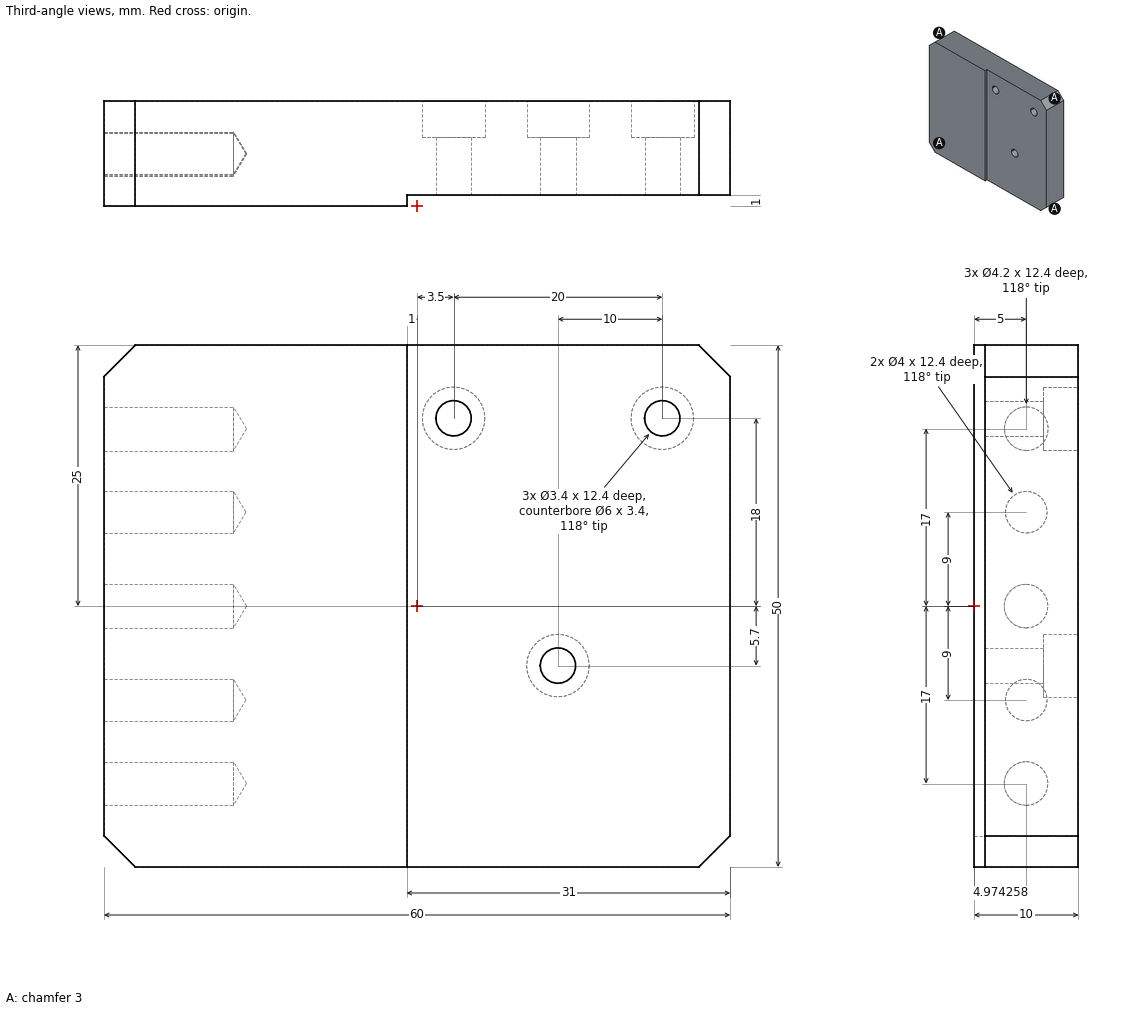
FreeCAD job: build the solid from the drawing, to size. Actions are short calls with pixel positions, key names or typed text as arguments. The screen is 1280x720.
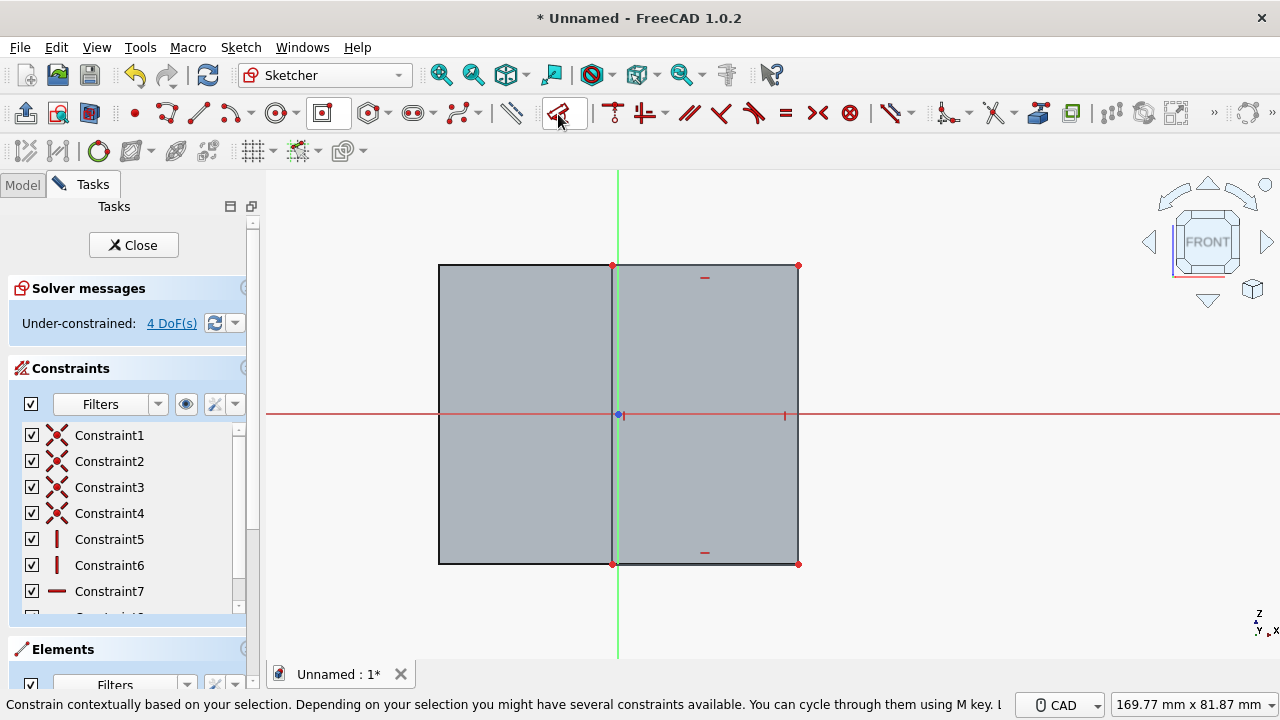
scroll(612, 355, up, 5)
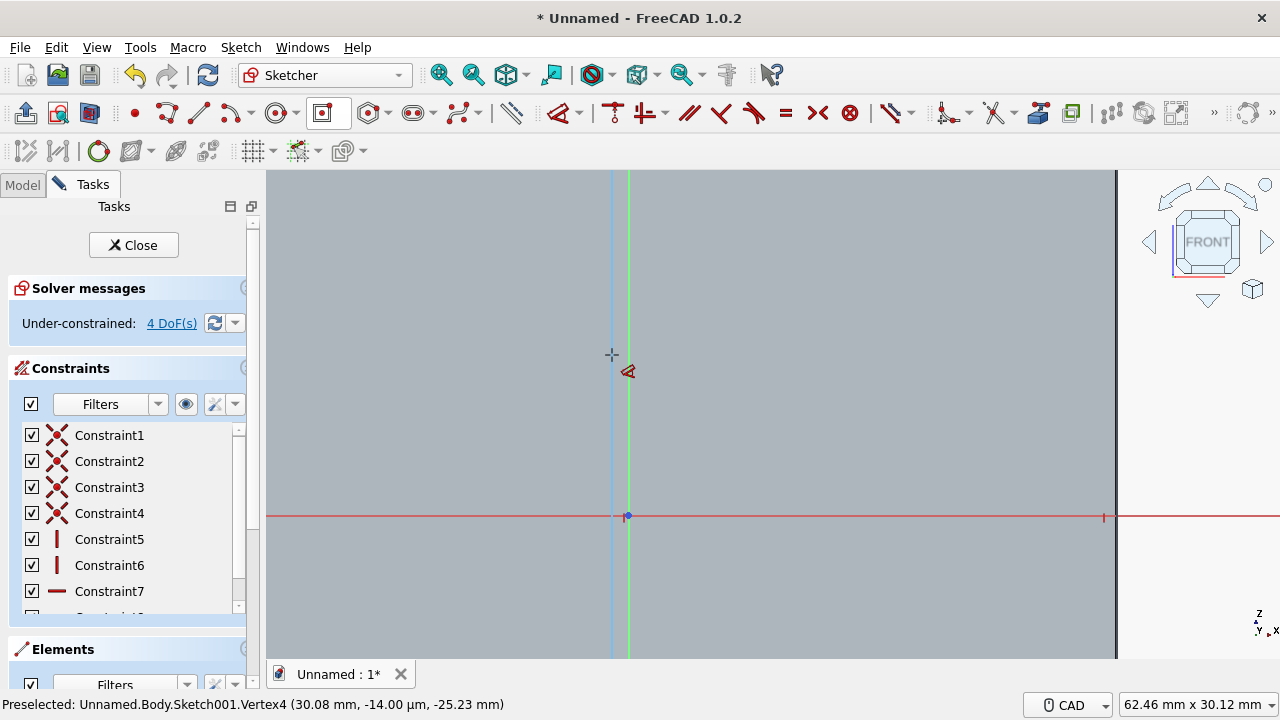
click(612, 355)
click(578, 414)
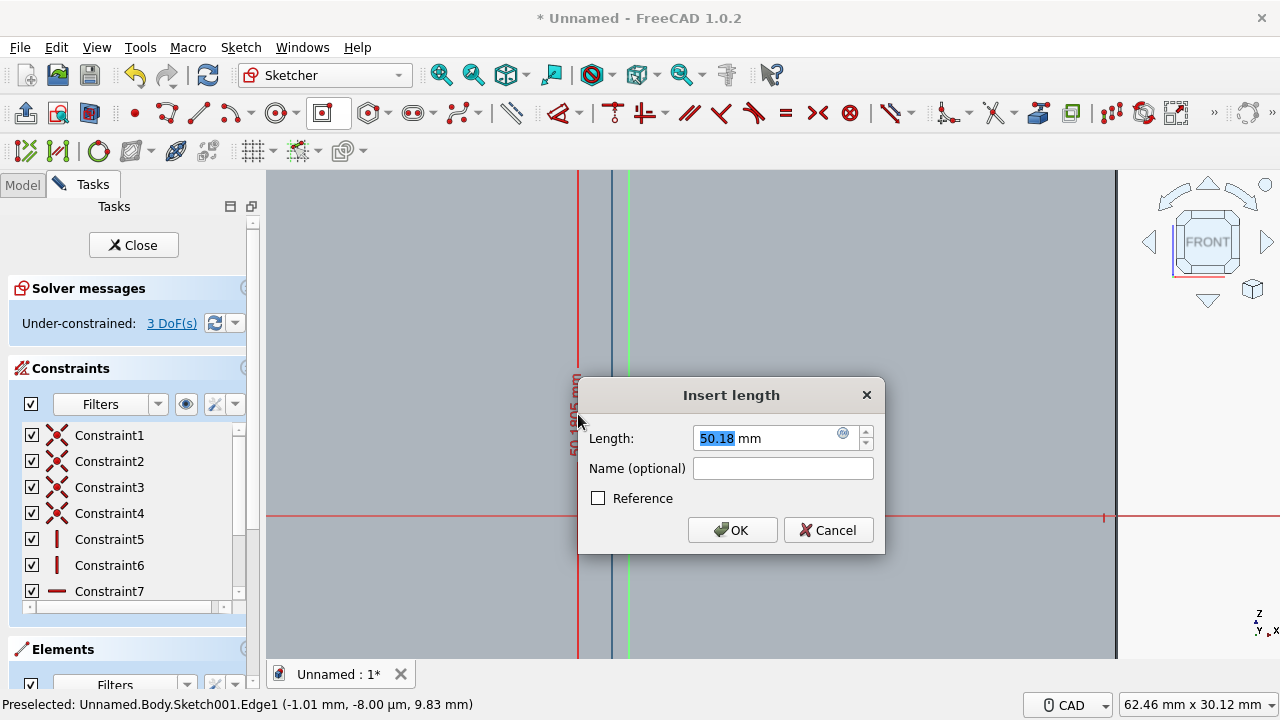
text(50)
key(Return)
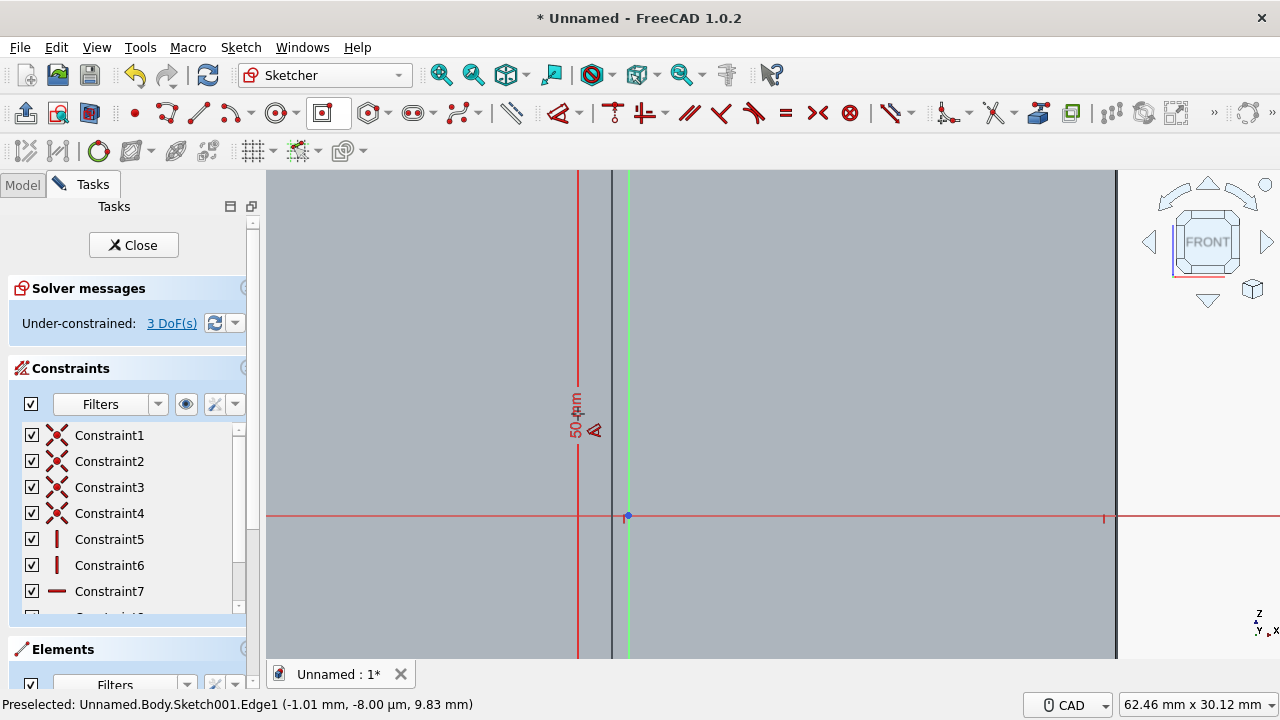
scroll(612, 356, down, 5)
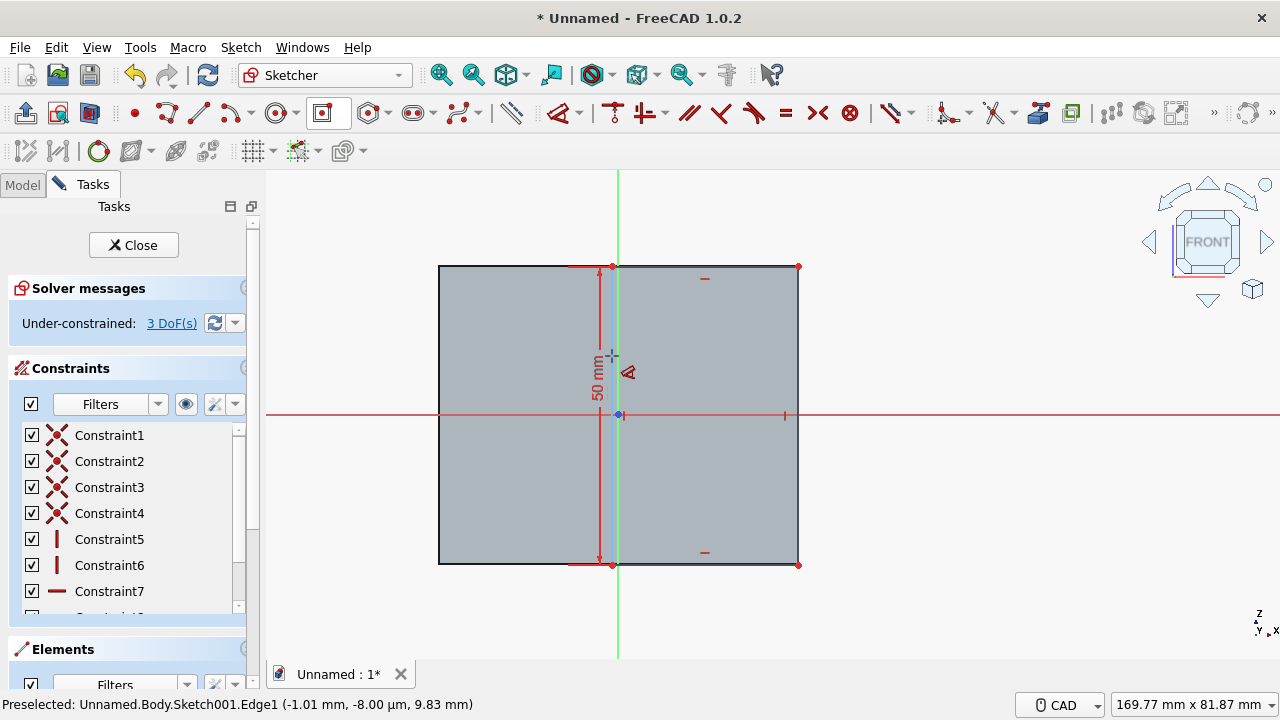
click(668, 565)
click(705, 599)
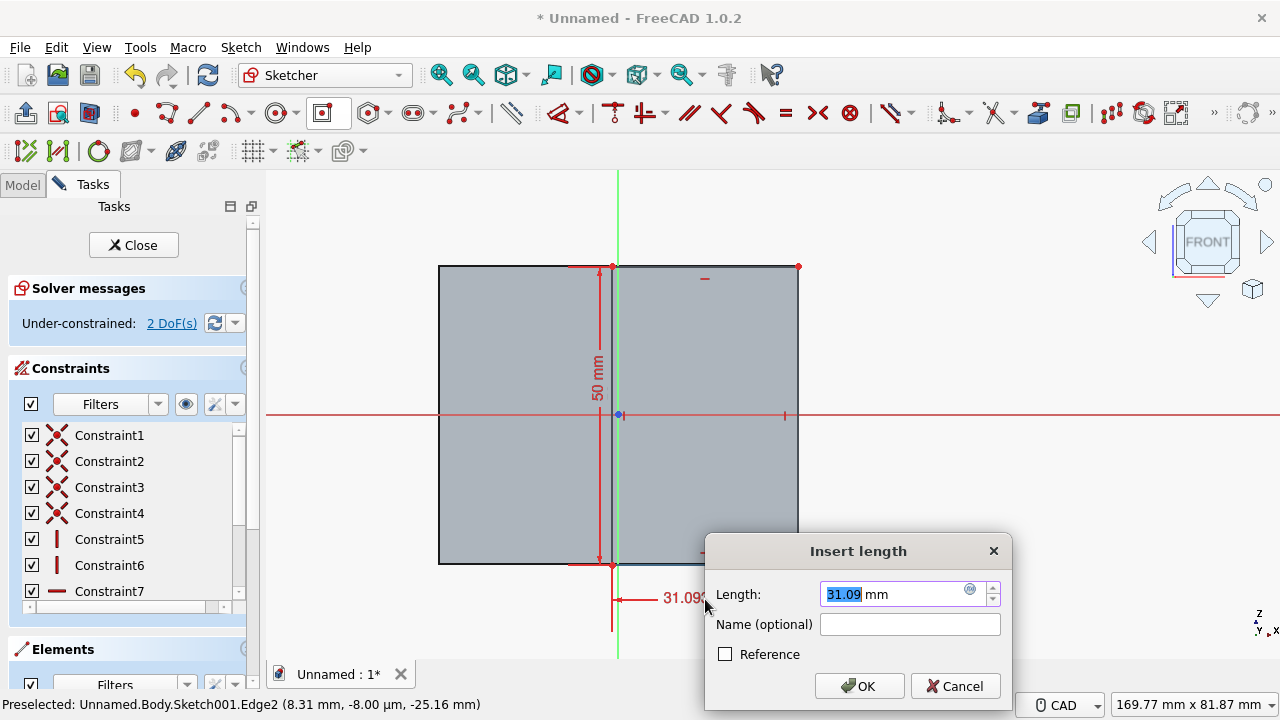
text(31)
key(Return)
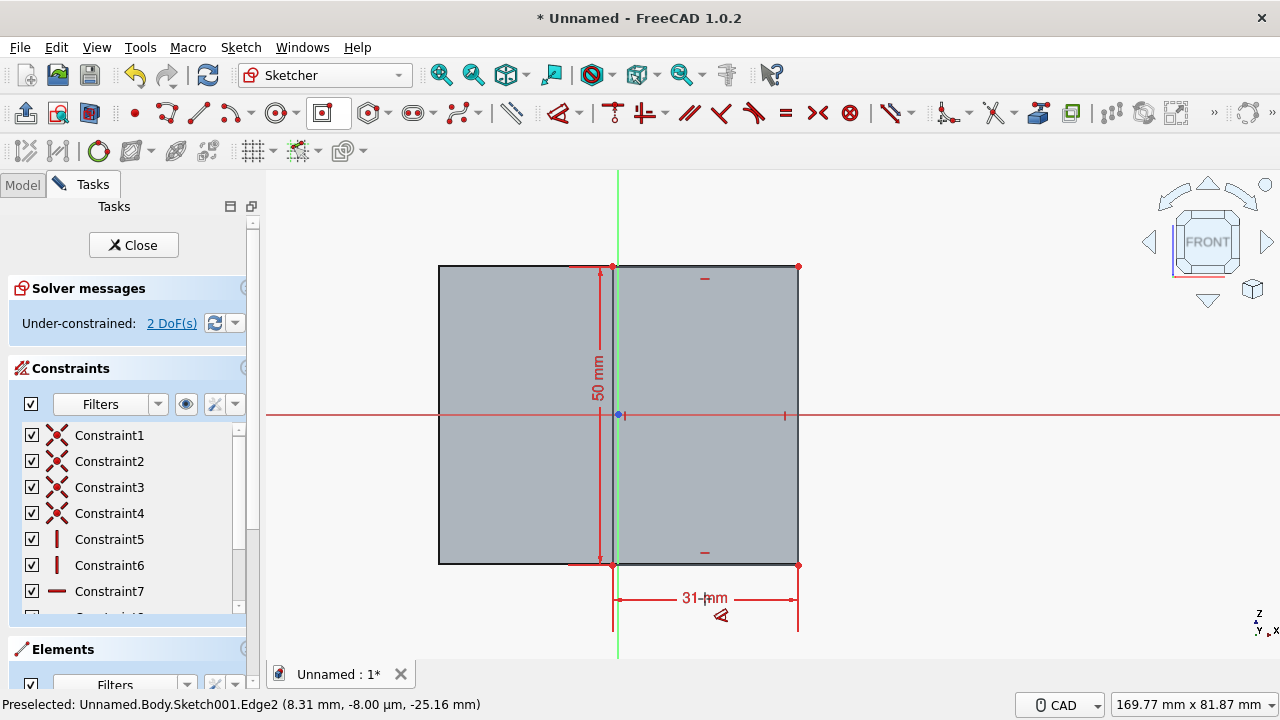
scroll(613, 267, up, 10)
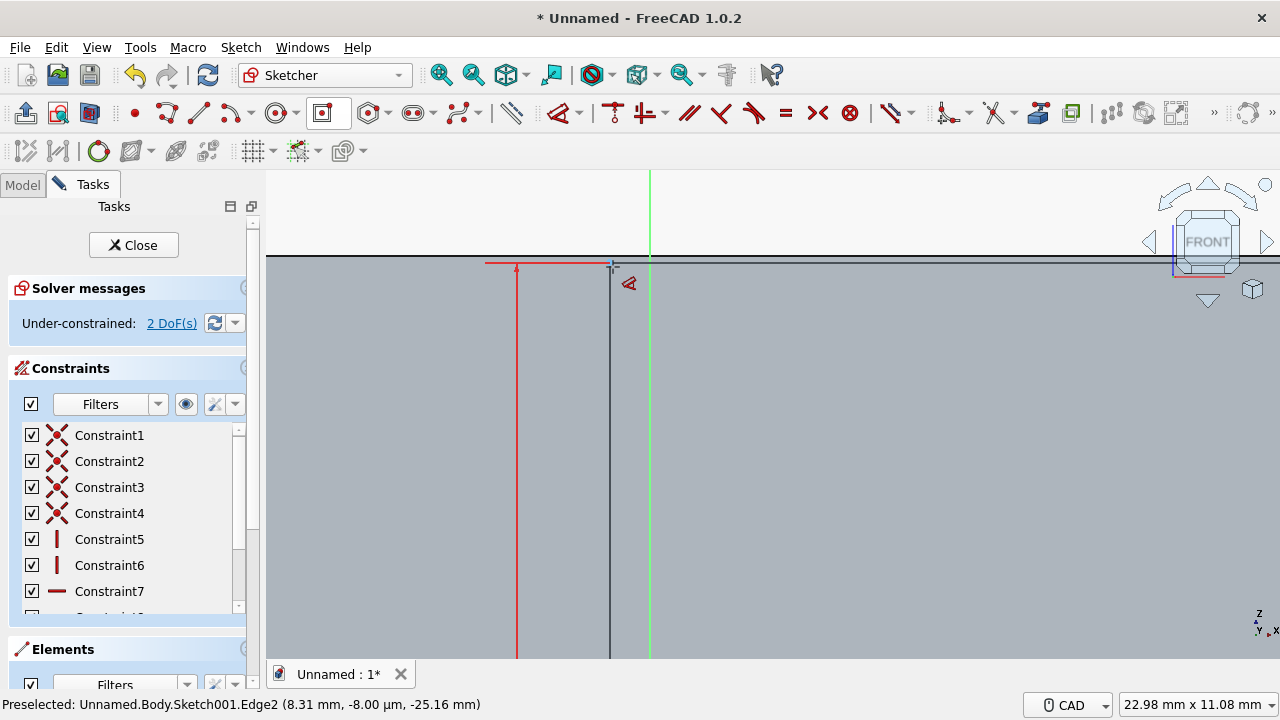
click(610, 263)
click(630, 229)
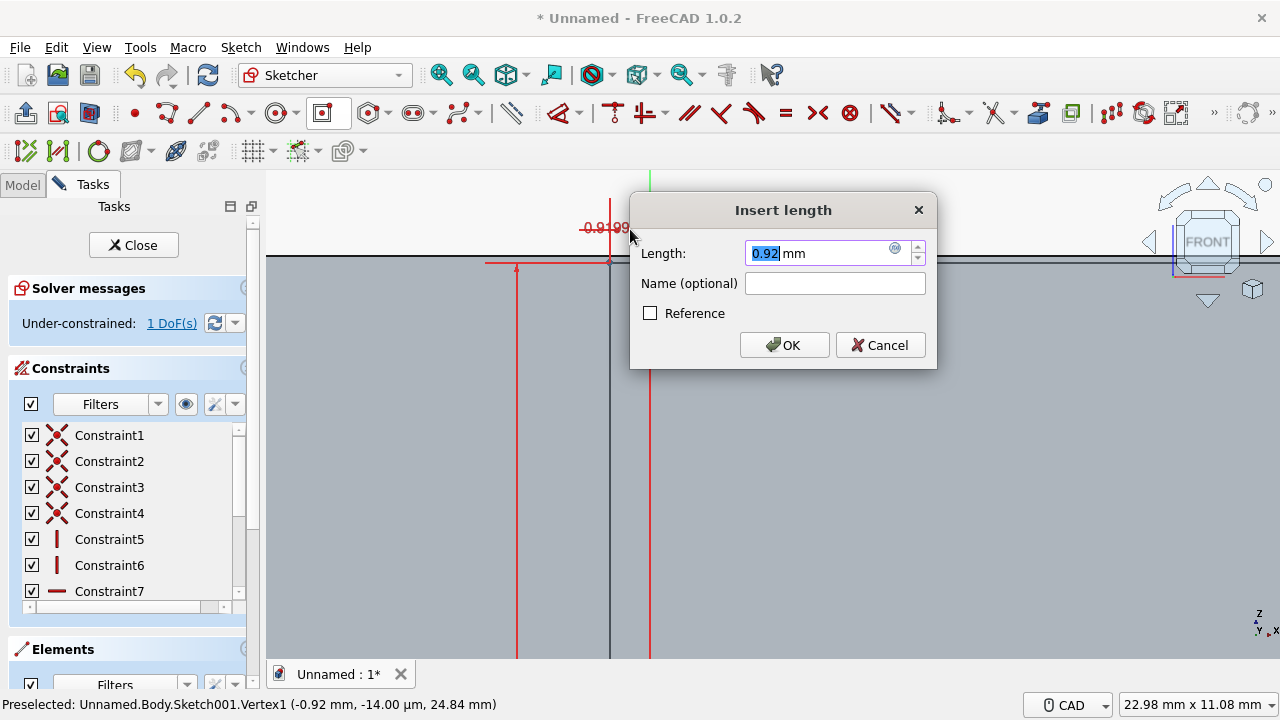
text(1)
key(Return)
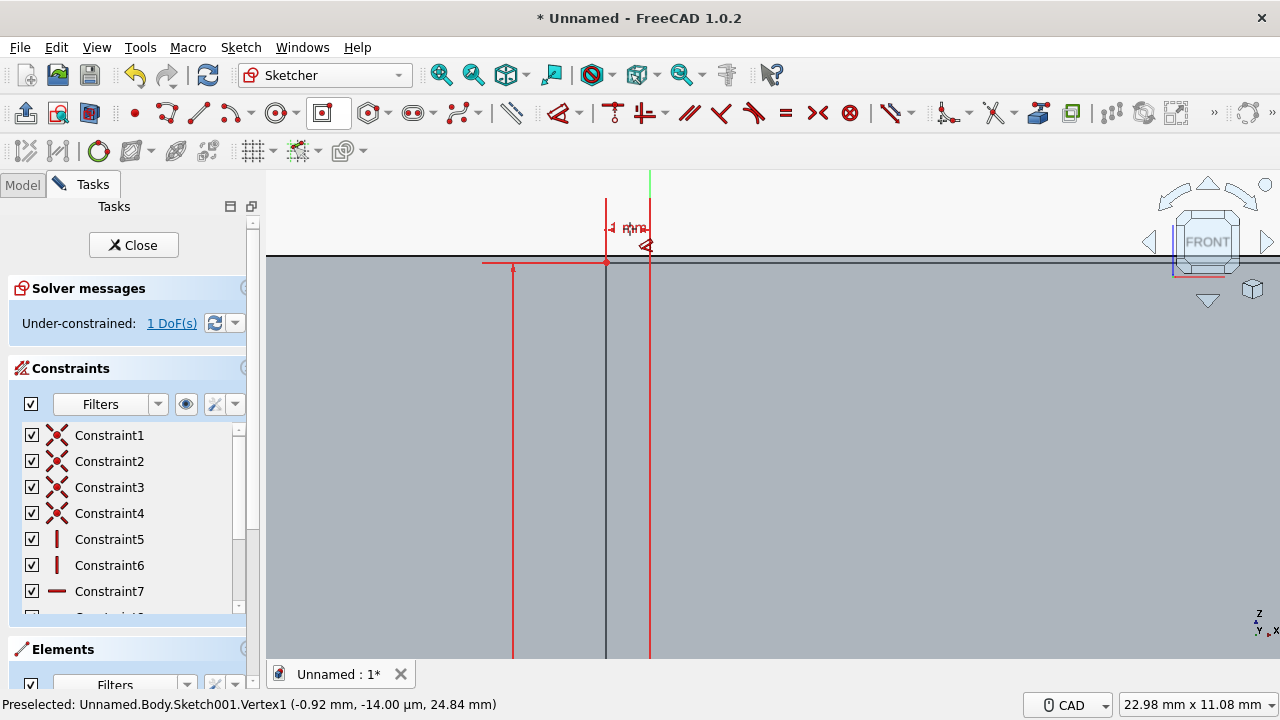
scroll(613, 267, down, 10)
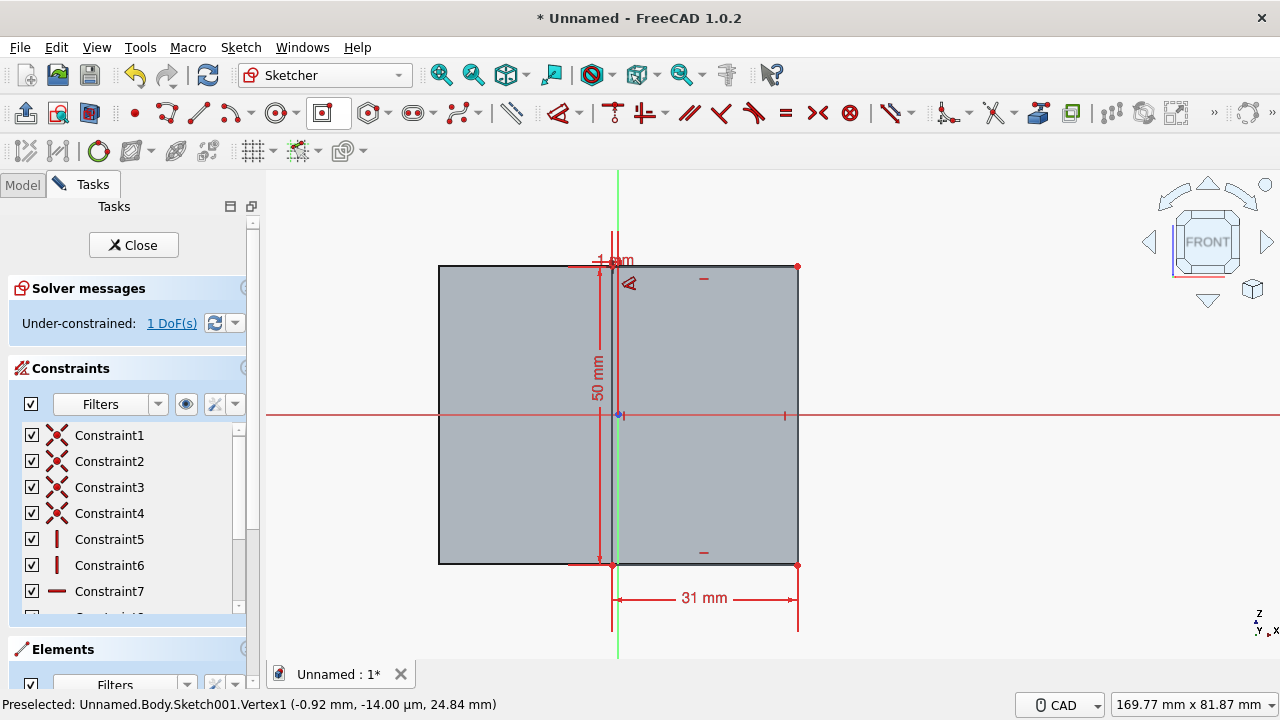
click(612, 267)
click(578, 341)